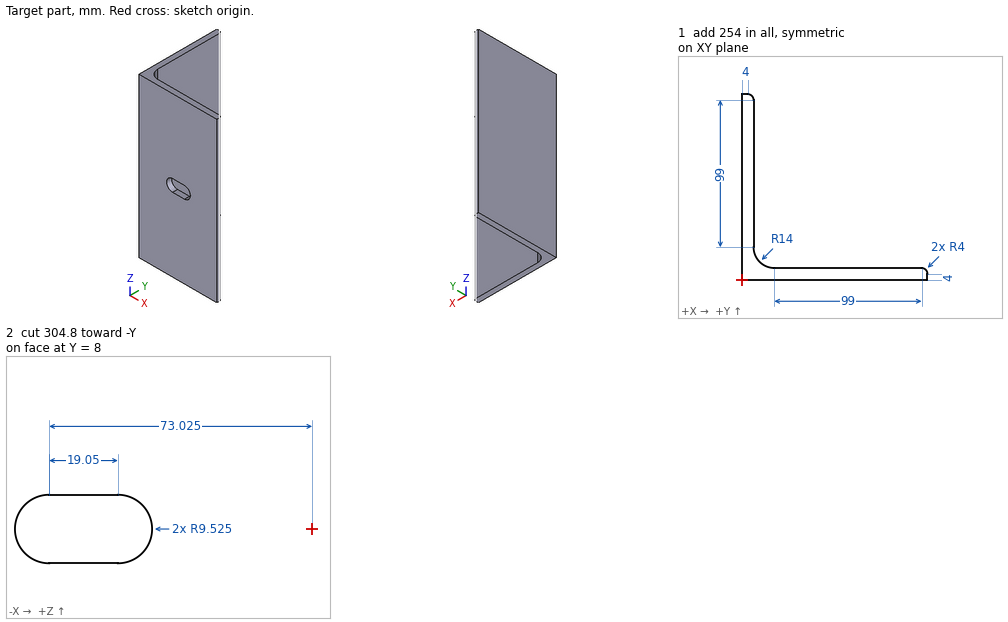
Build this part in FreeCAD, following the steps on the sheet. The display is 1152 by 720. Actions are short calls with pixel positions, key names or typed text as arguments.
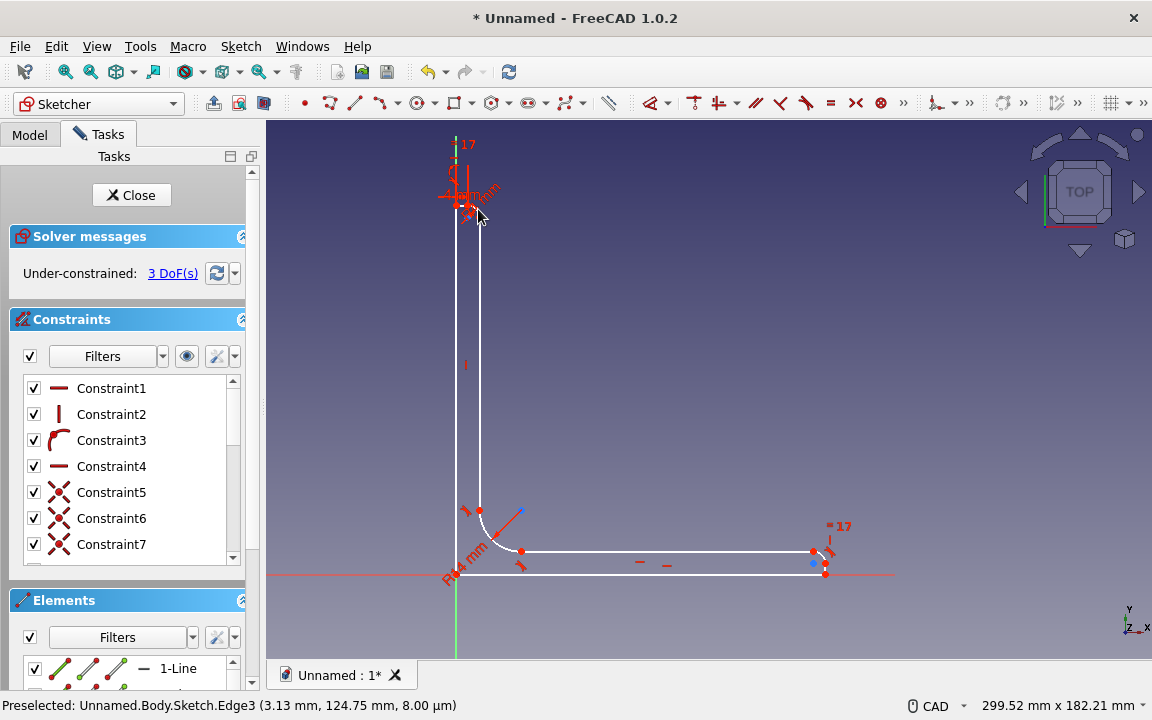
scroll(825, 571, up, 8)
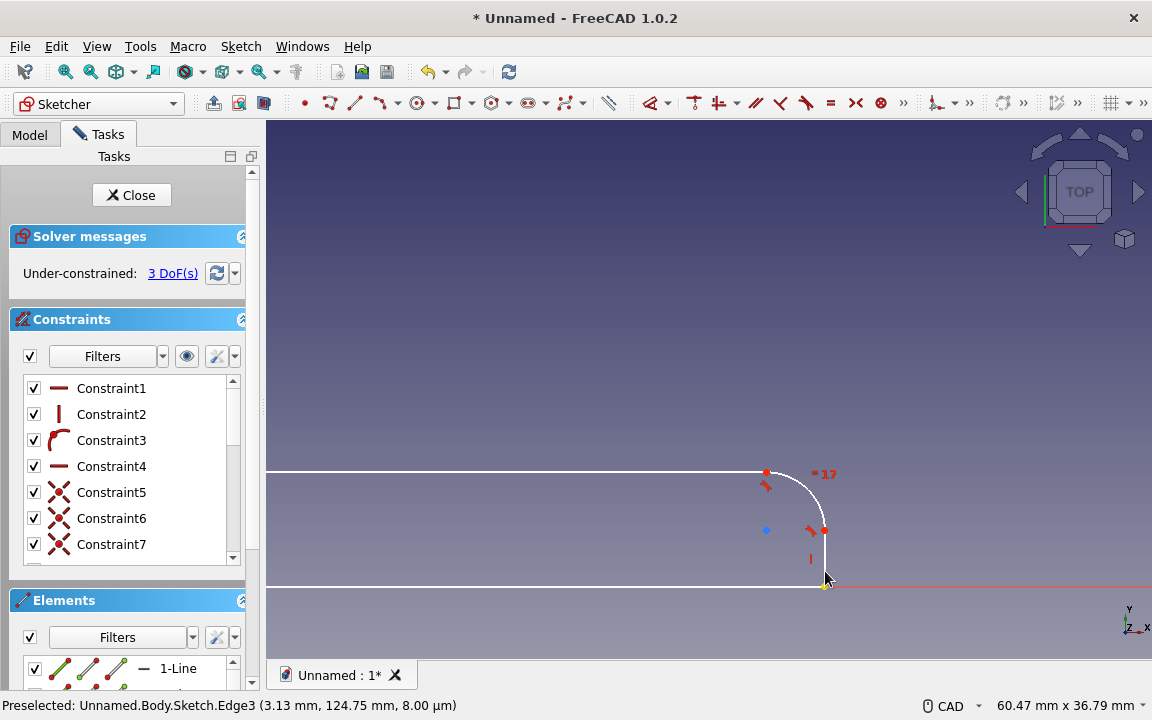
click(825, 570)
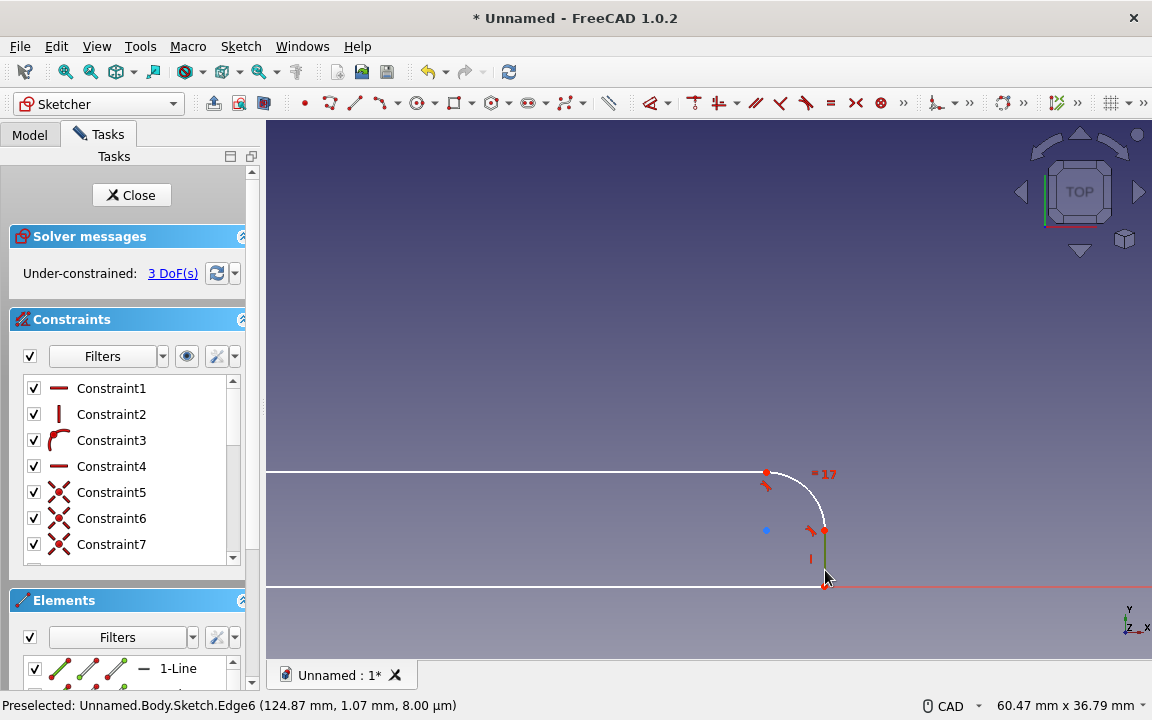
click(668, 104)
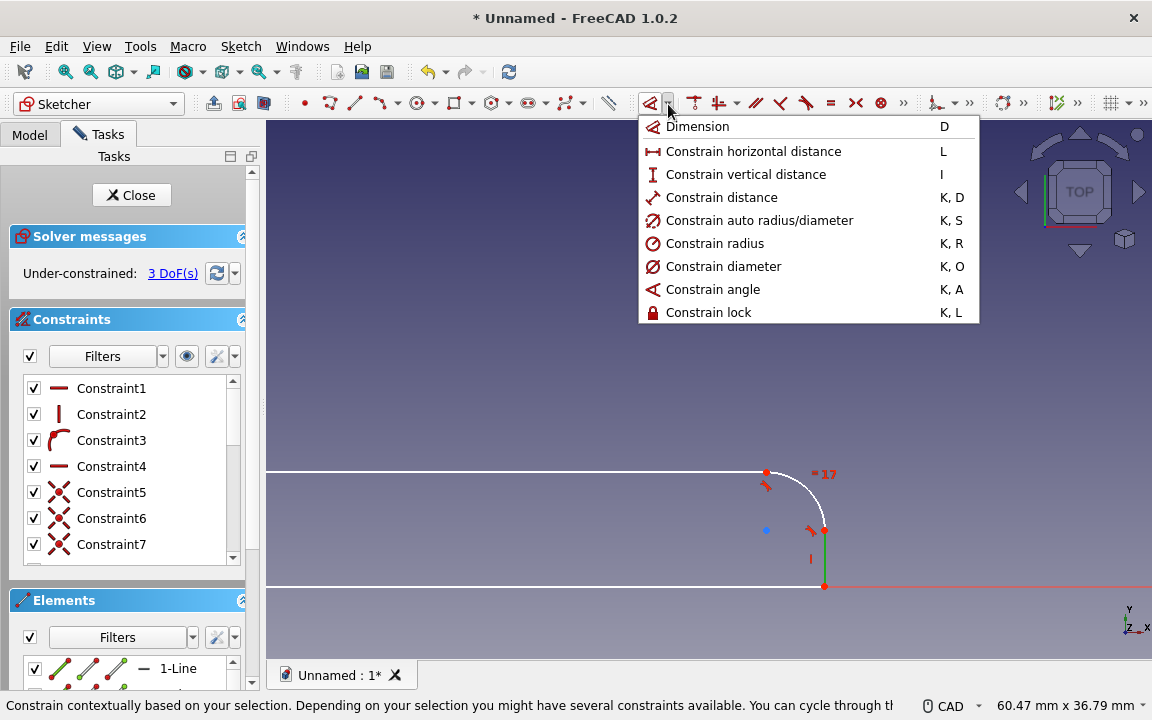
click(809, 174)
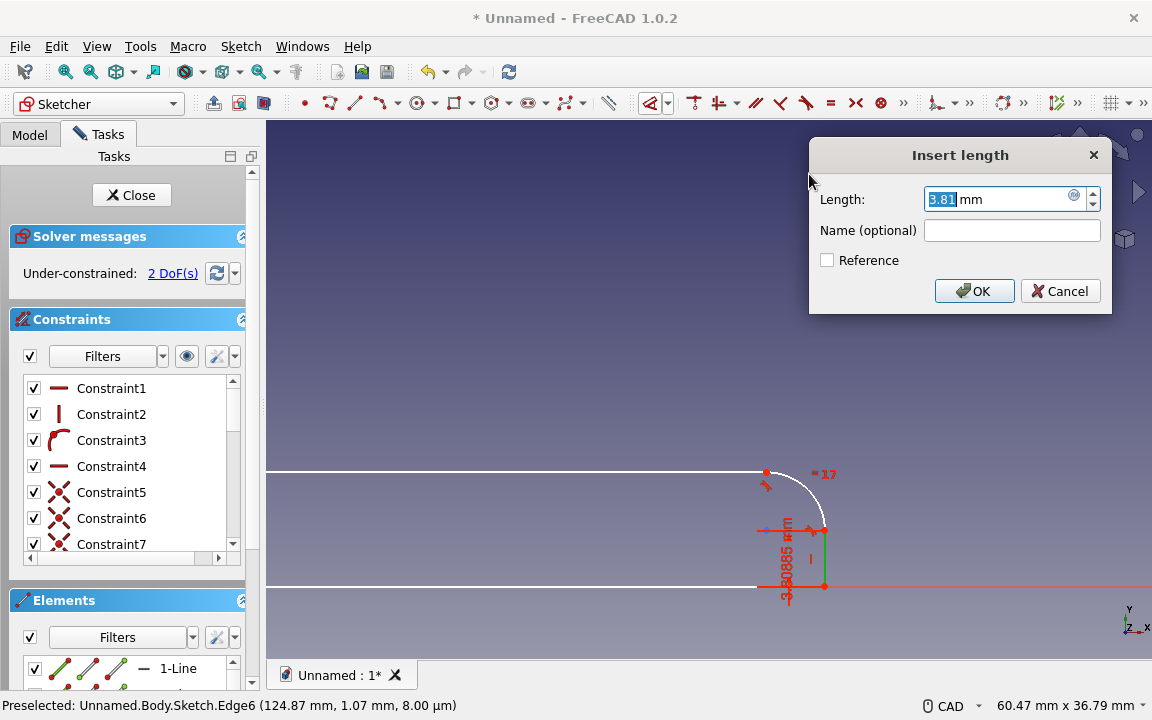
text(4)
key(Return)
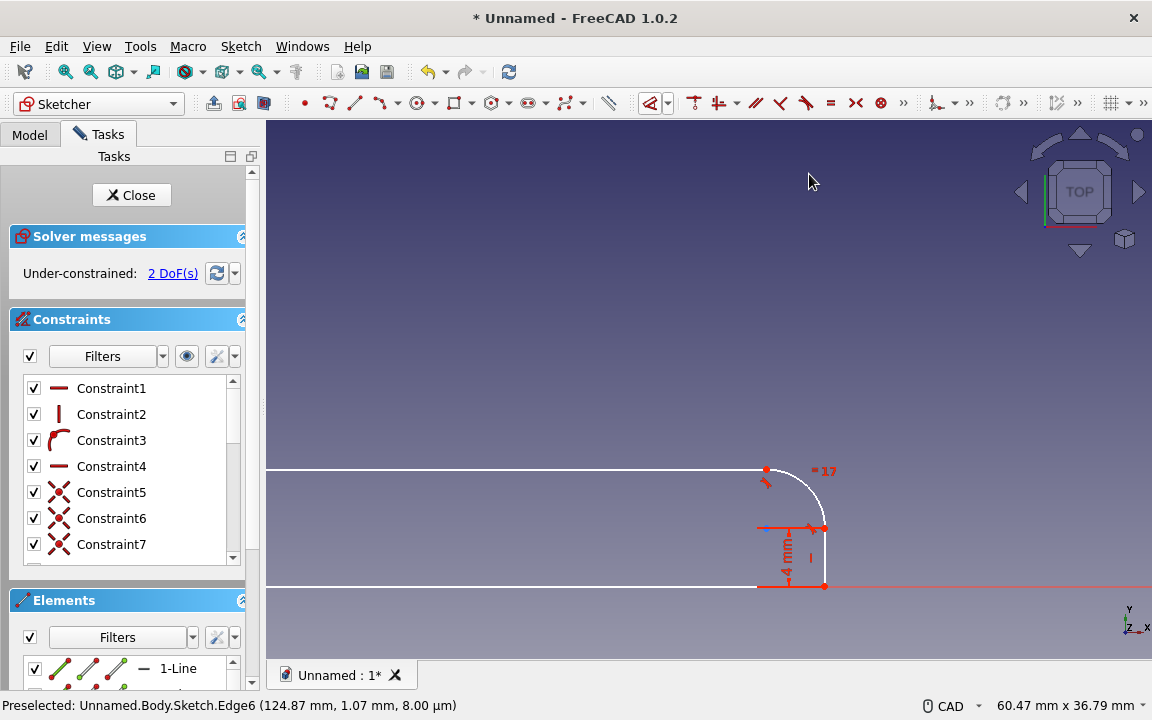
scroll(825, 571, down, 8)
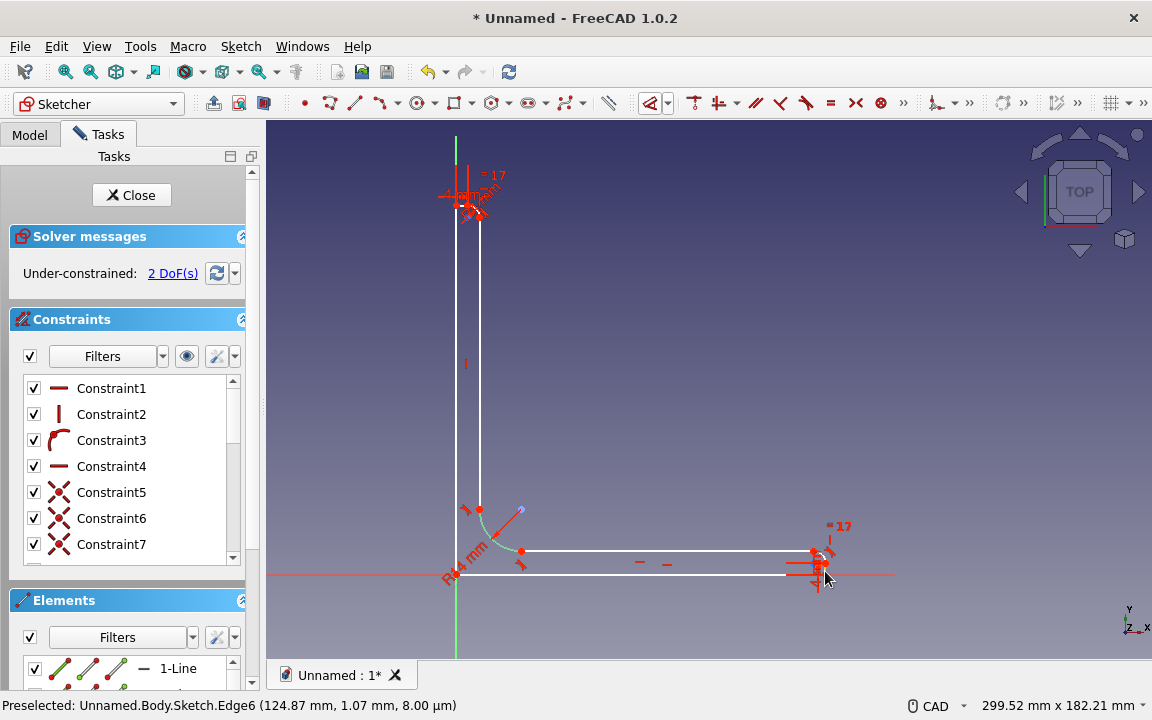
click(726, 551)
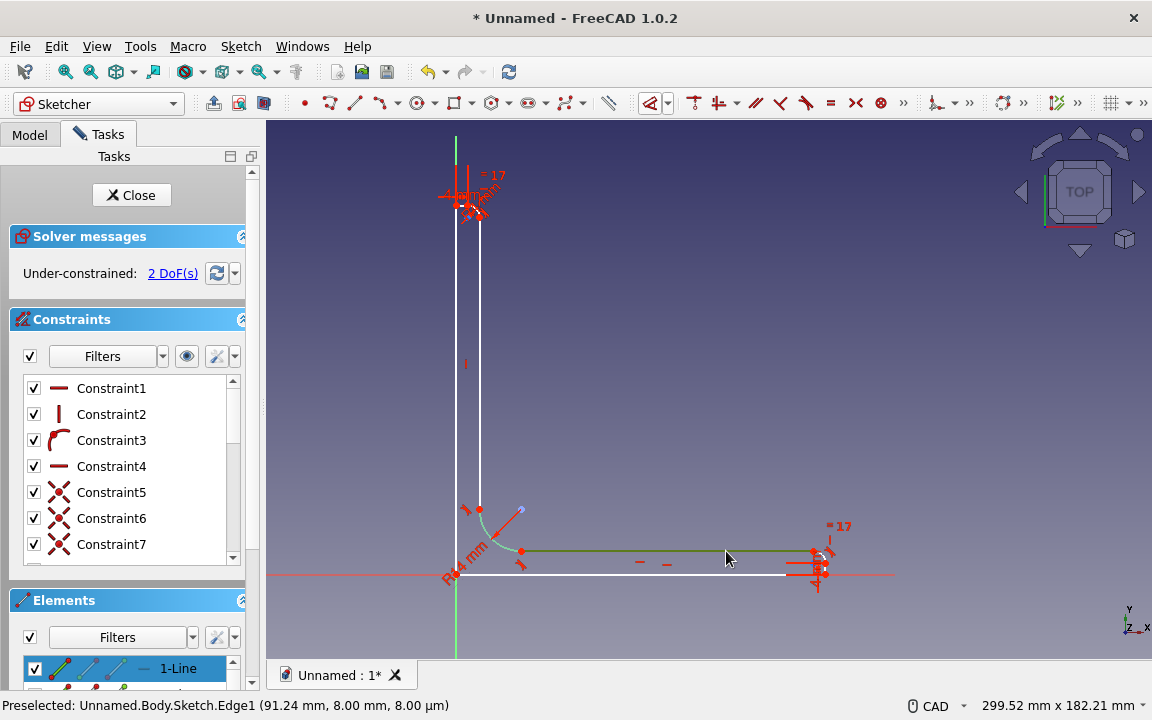
click(668, 104)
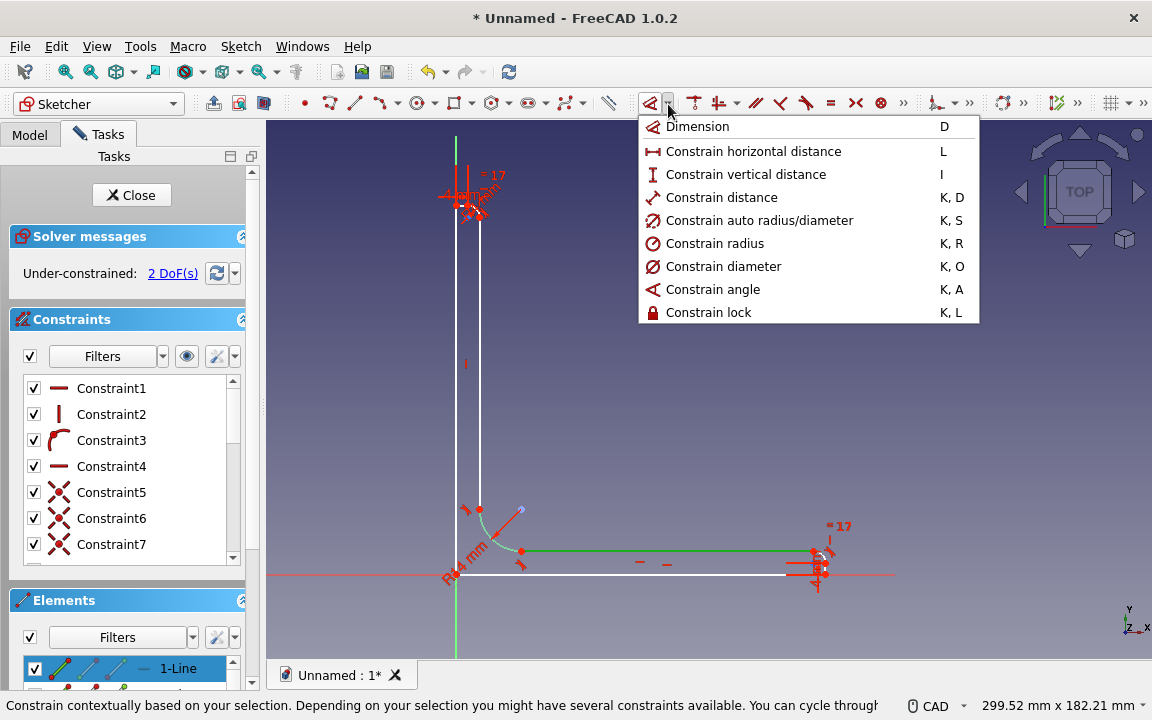
click(809, 152)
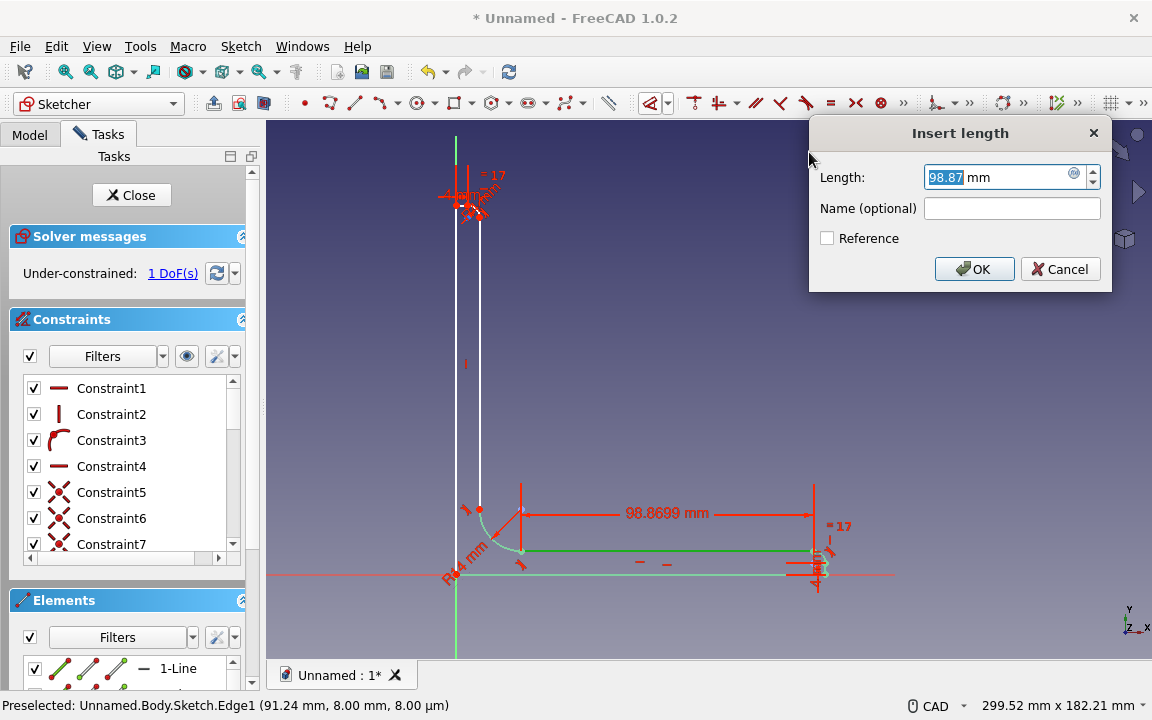
text(99)
key(Return)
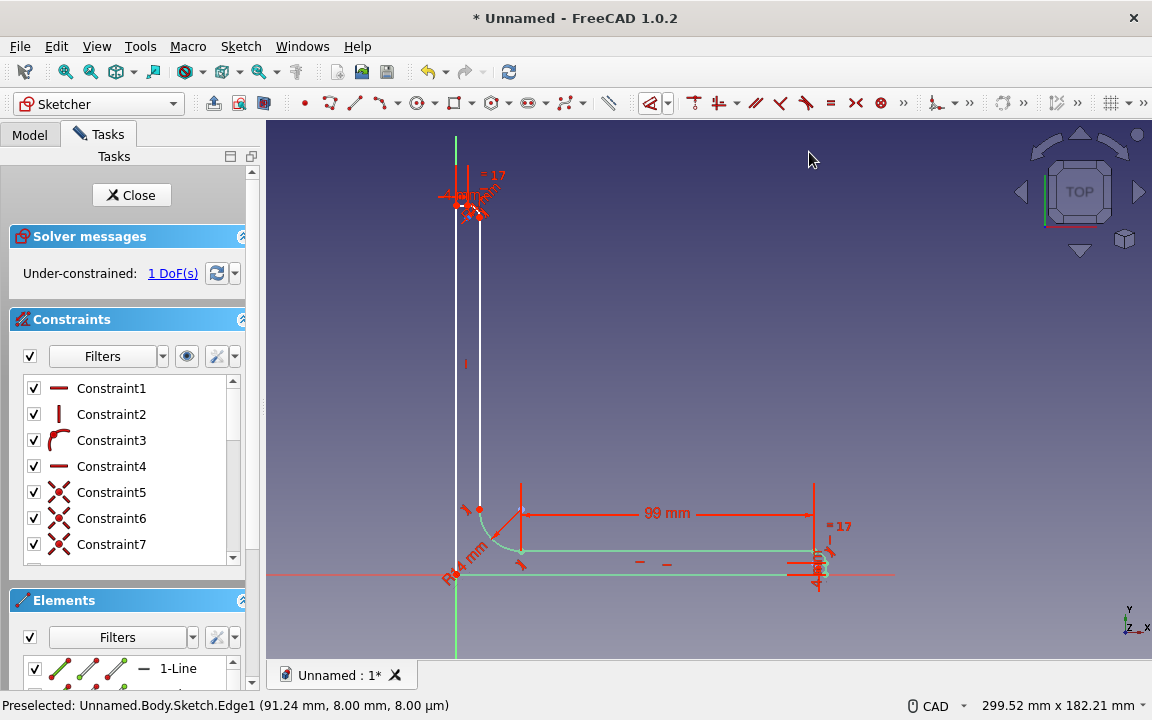
click(480, 422)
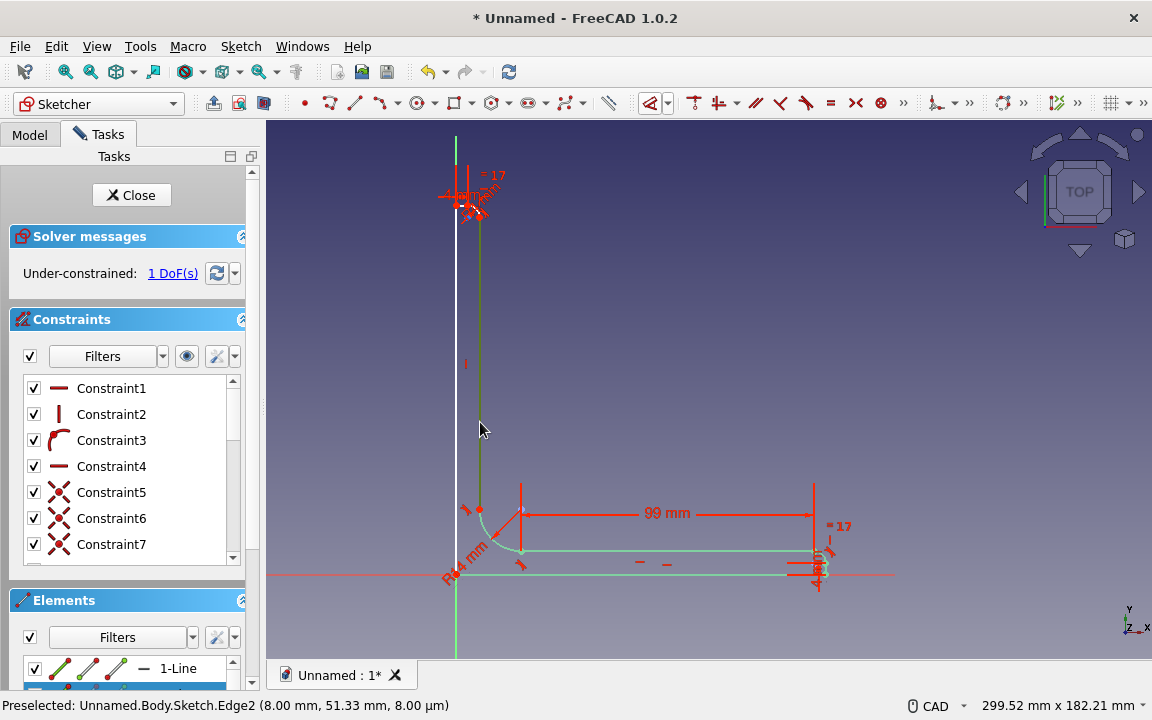
key(i)